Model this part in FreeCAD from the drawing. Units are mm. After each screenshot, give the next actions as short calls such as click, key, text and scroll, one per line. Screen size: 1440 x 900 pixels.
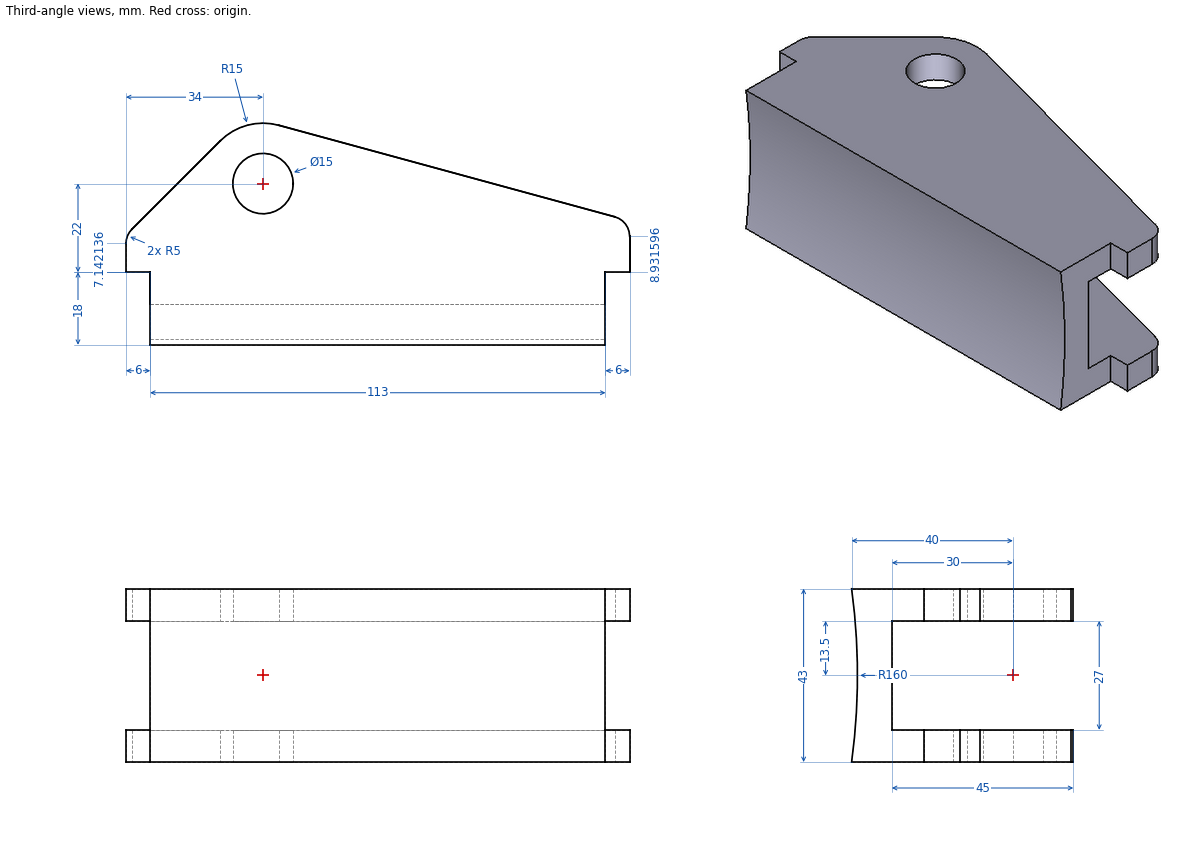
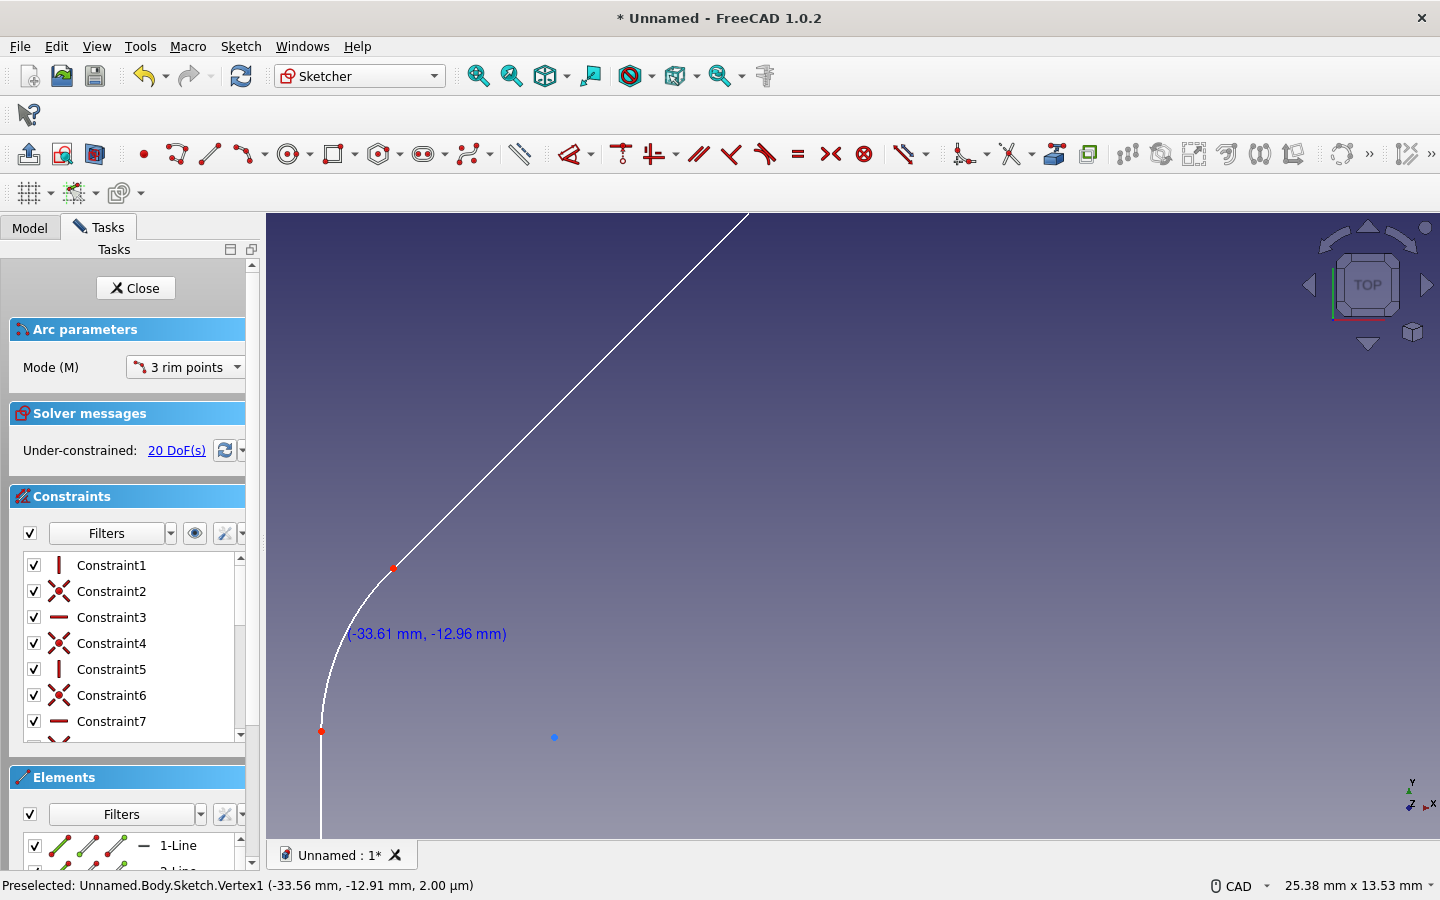
click(288, 154)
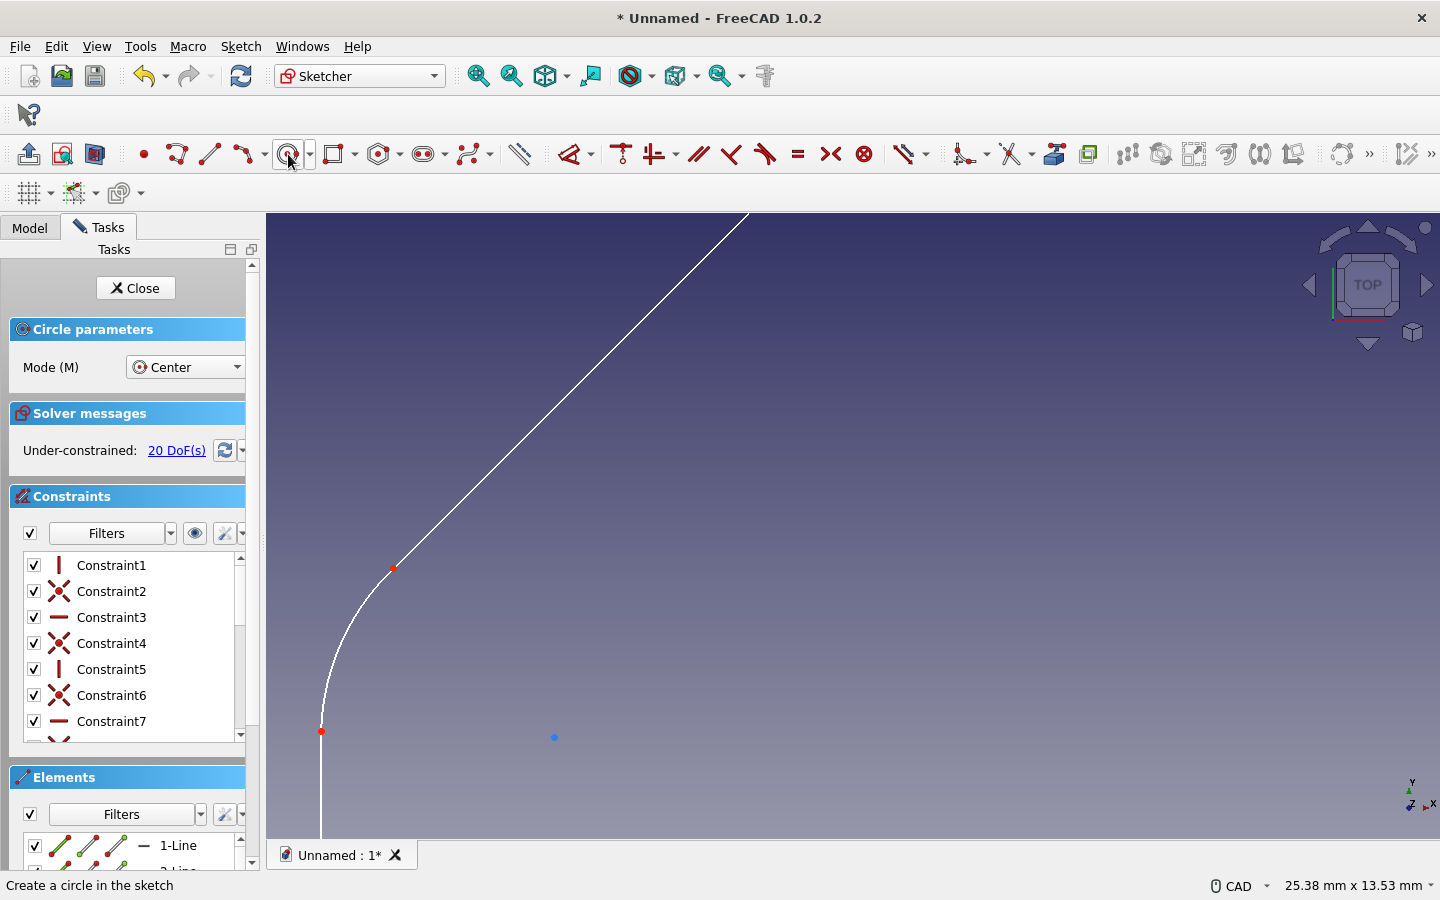
scroll(482, 513, down, 11)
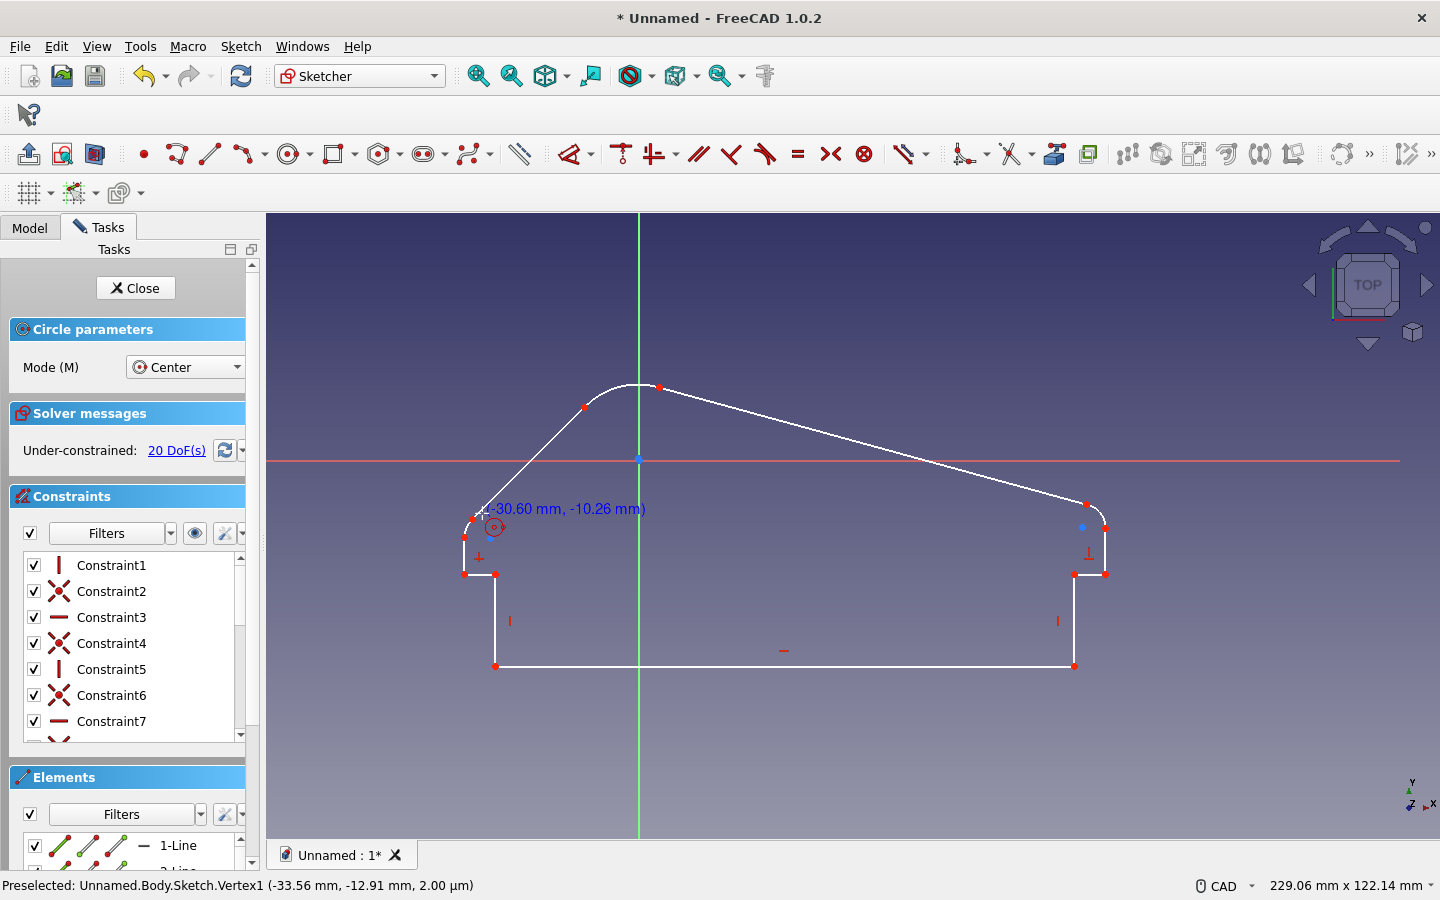
click(639, 461)
move(666, 434)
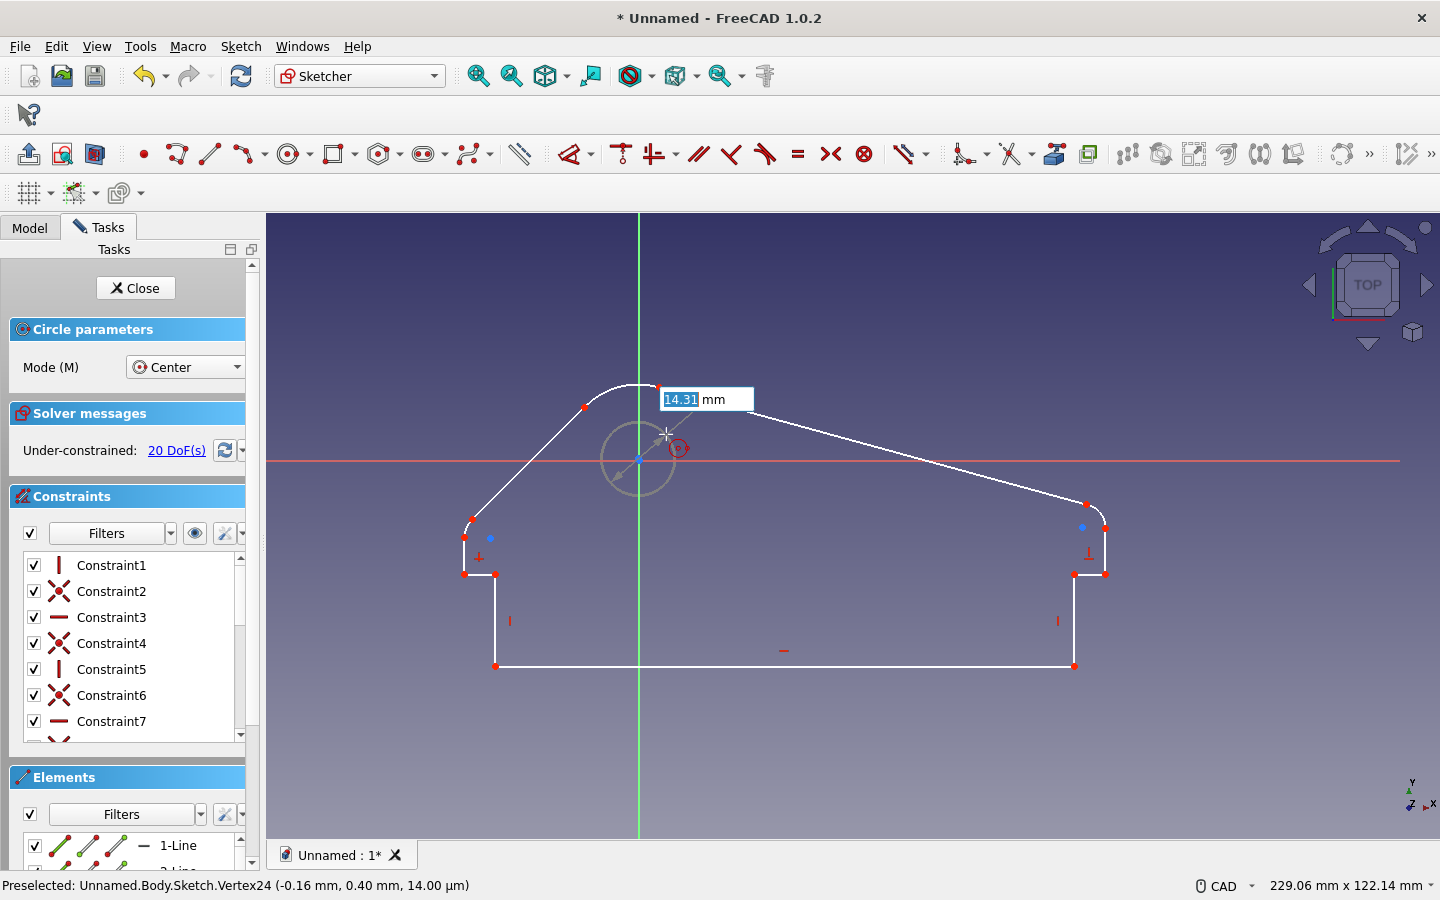
text(15)
key(Return)
key(Escape)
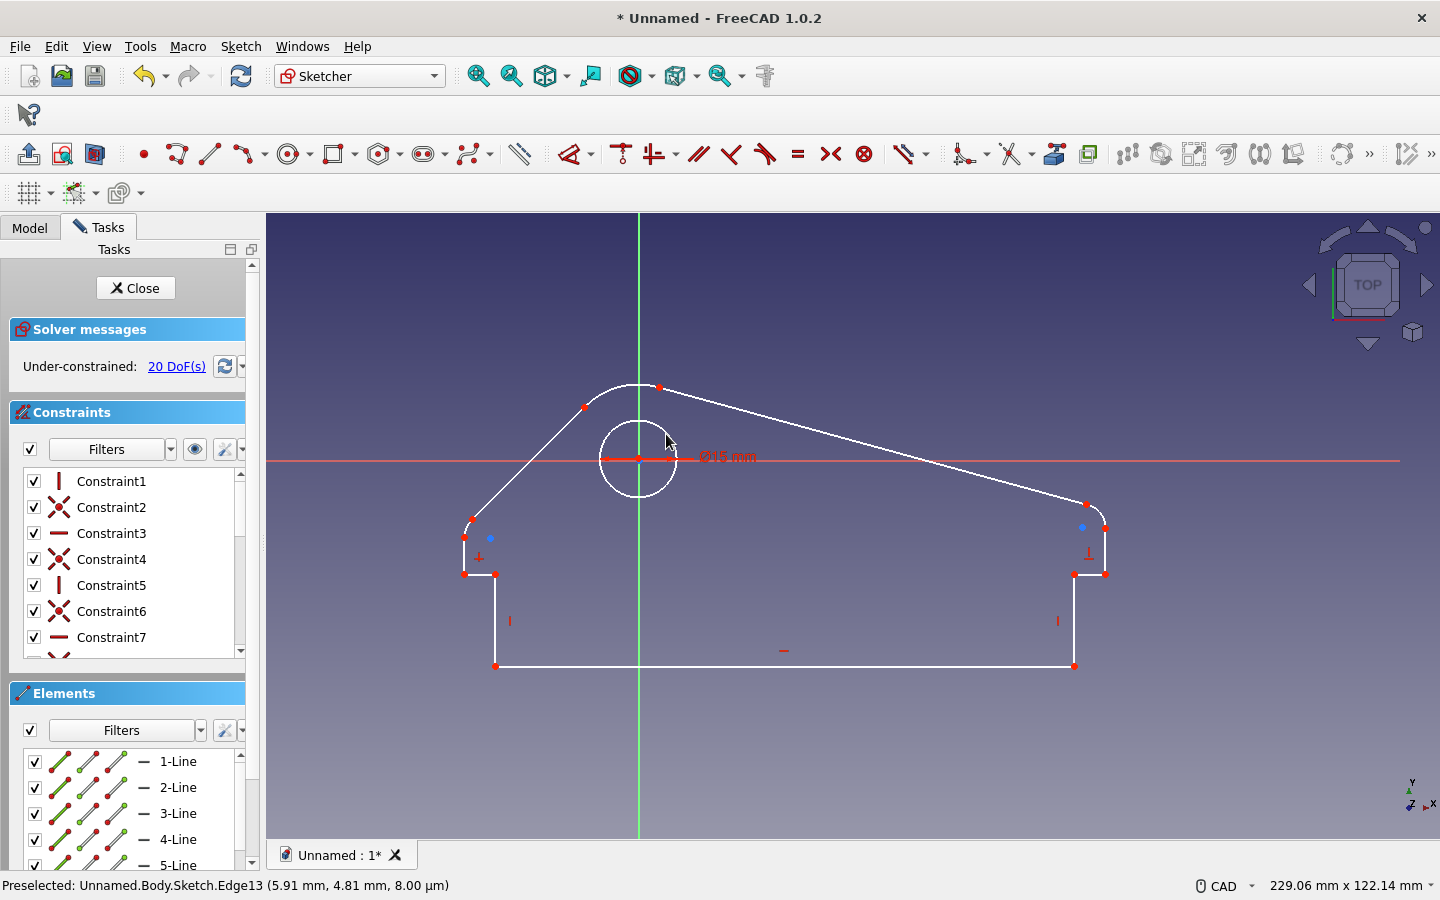
scroll(464, 549, up, 2)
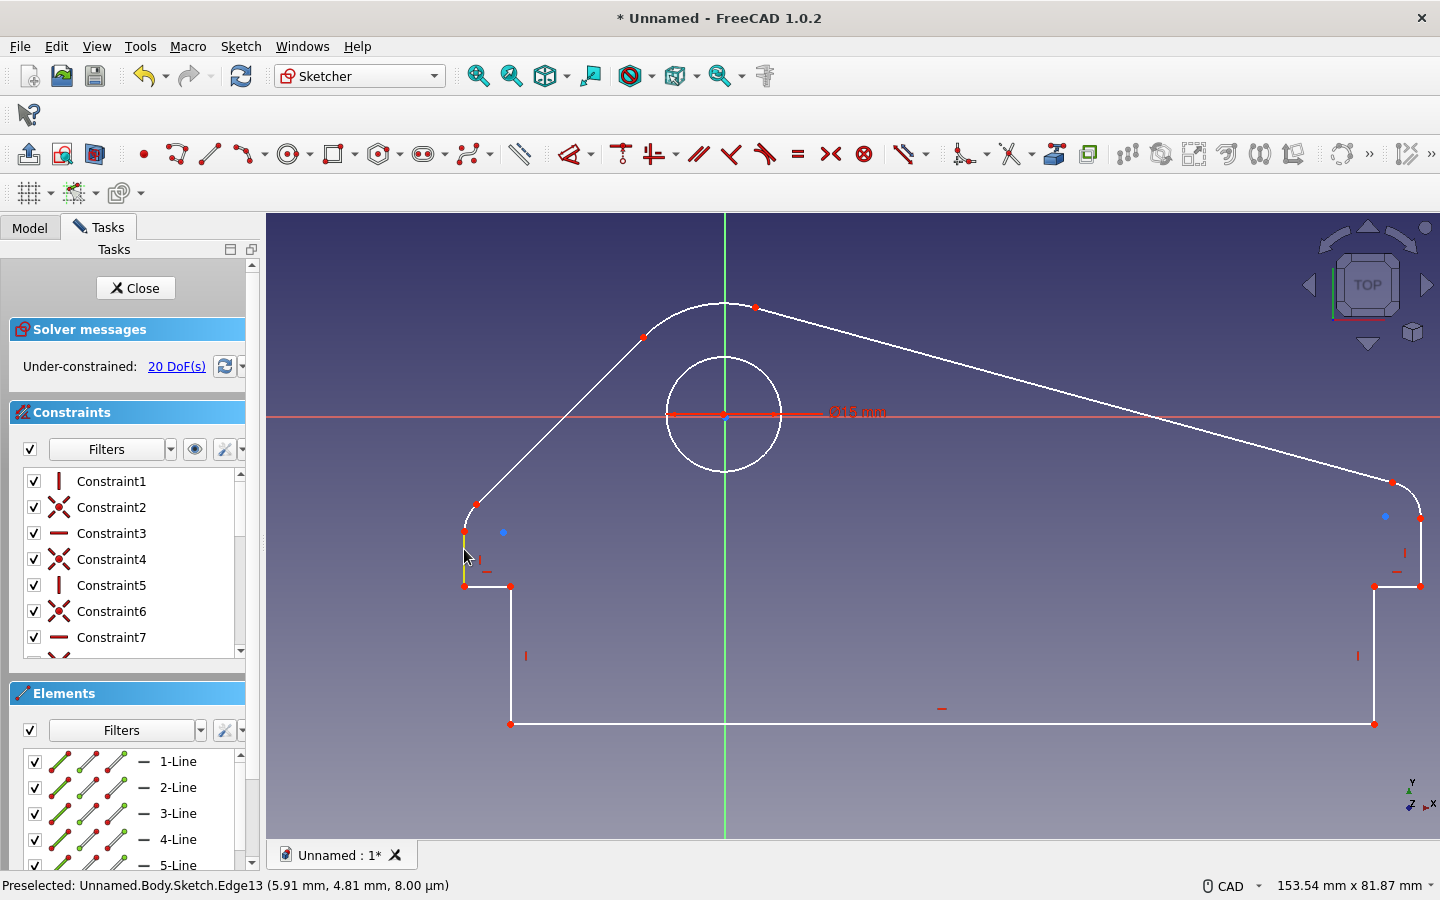
click(464, 548)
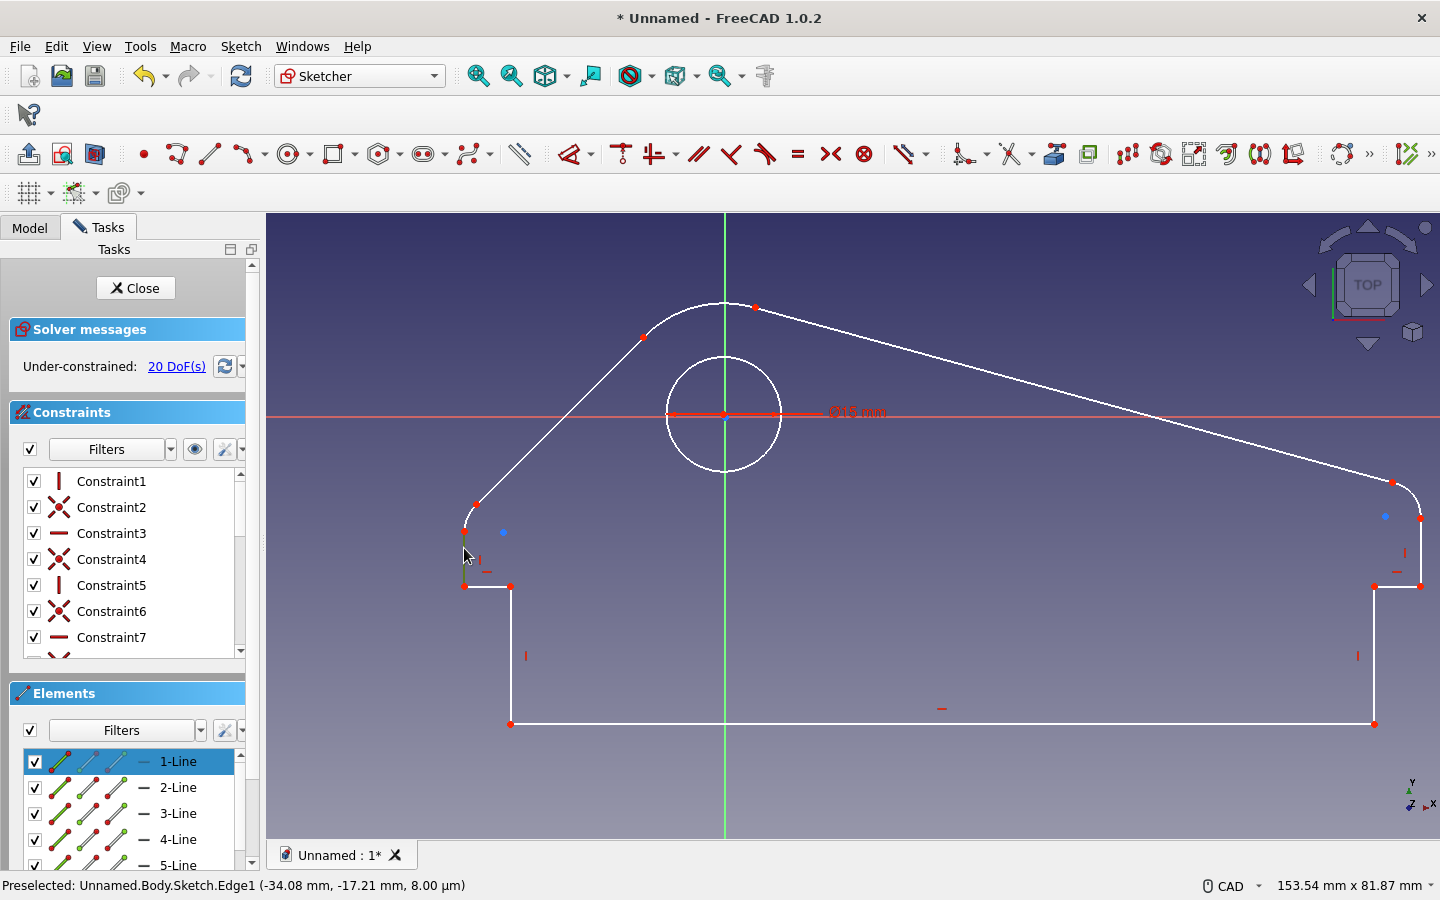
scroll(471, 512, up, 3)